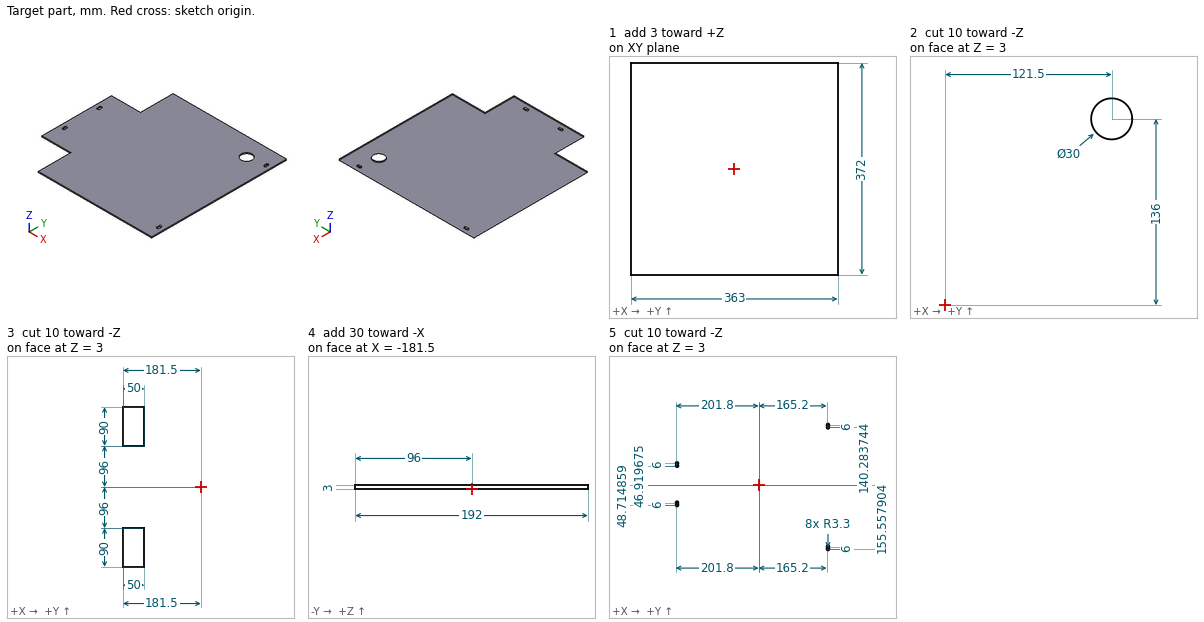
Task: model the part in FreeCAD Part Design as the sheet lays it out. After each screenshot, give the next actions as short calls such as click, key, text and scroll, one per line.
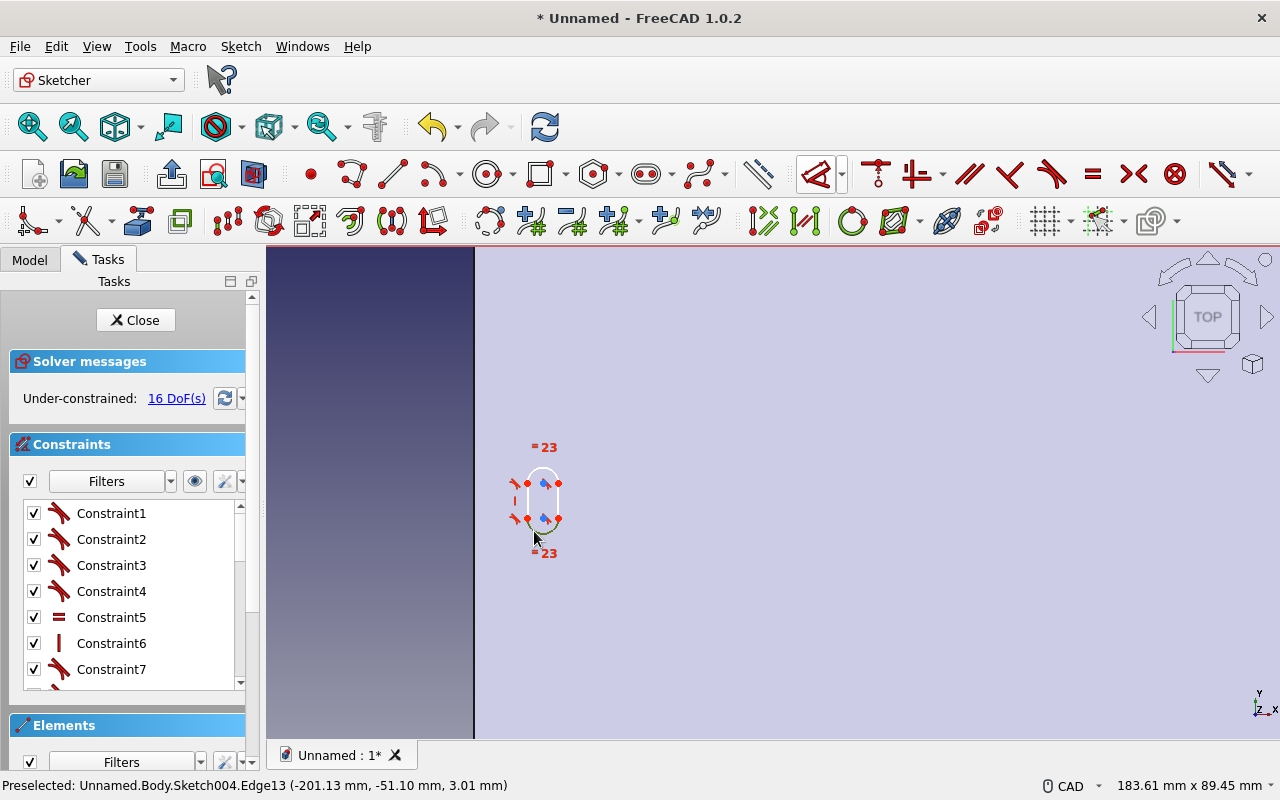
key(e)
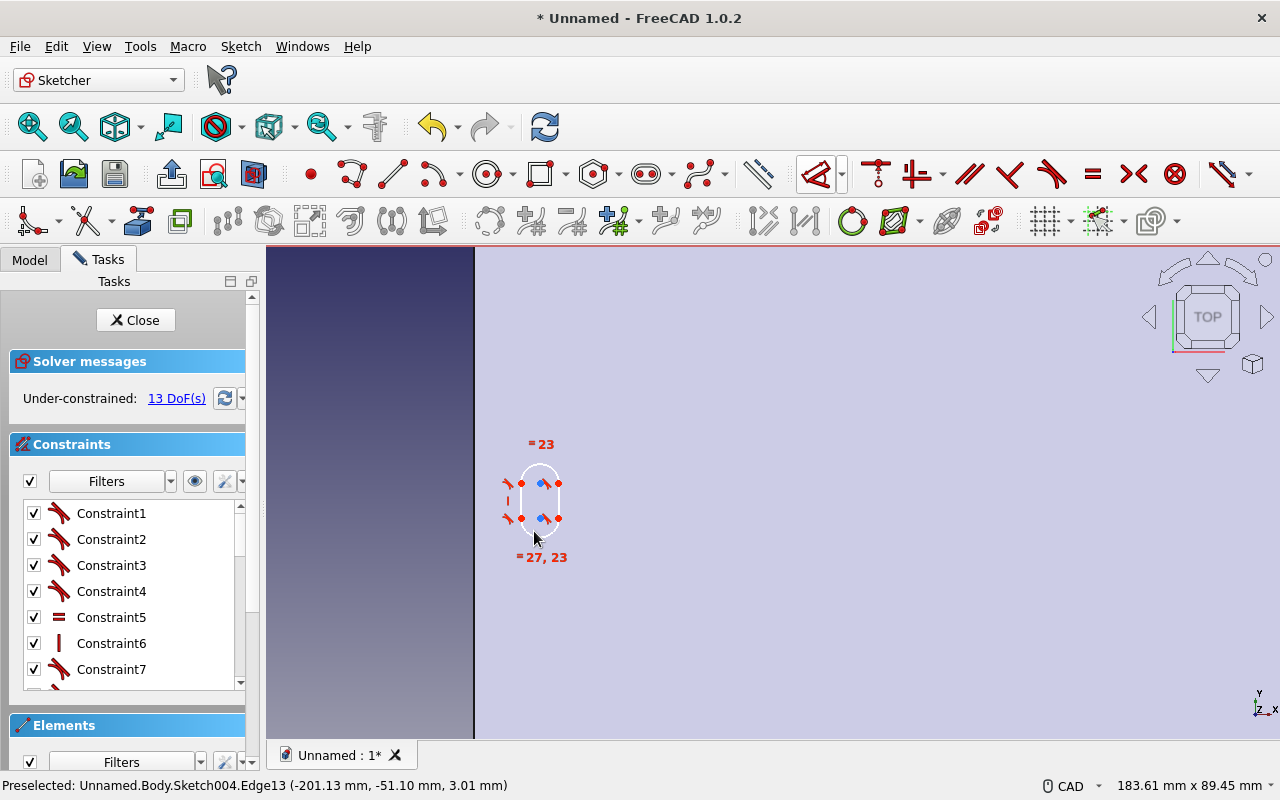
scroll(535, 536, down, 9)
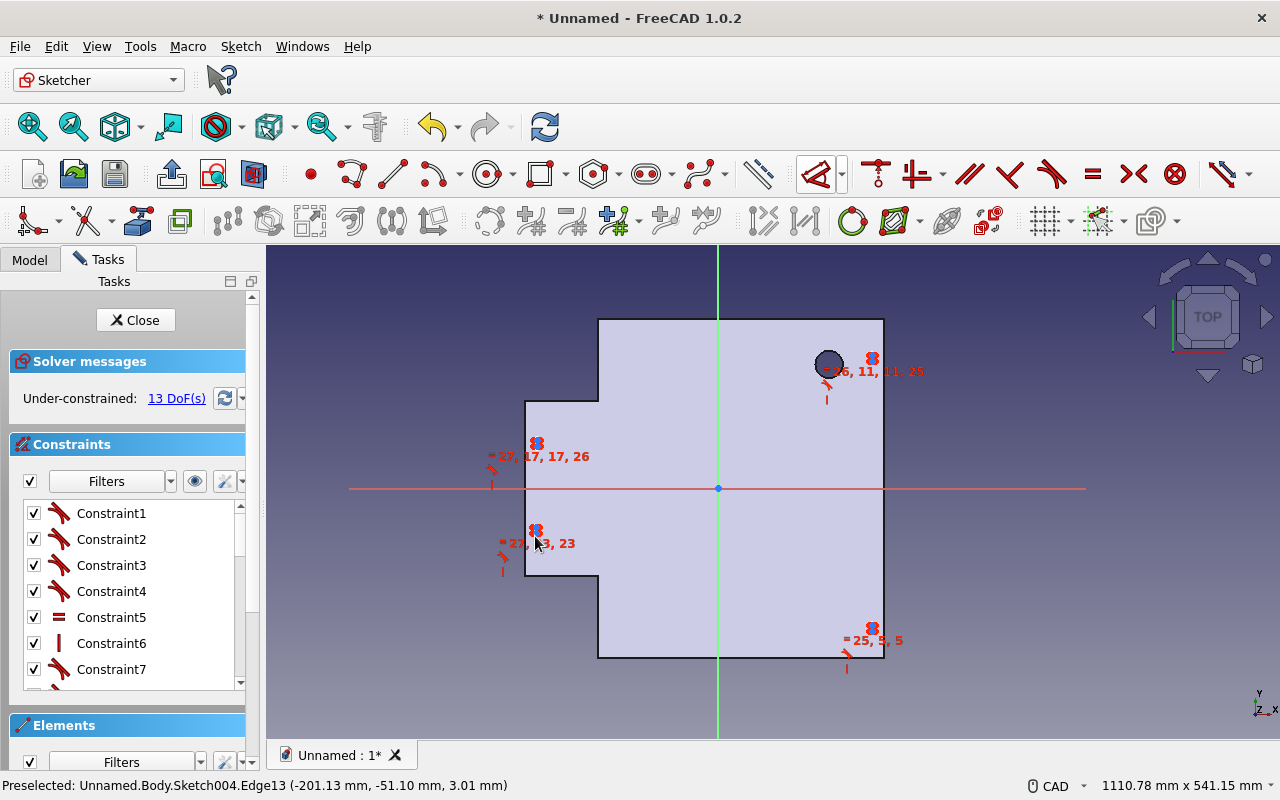
scroll(870, 634, up, 13)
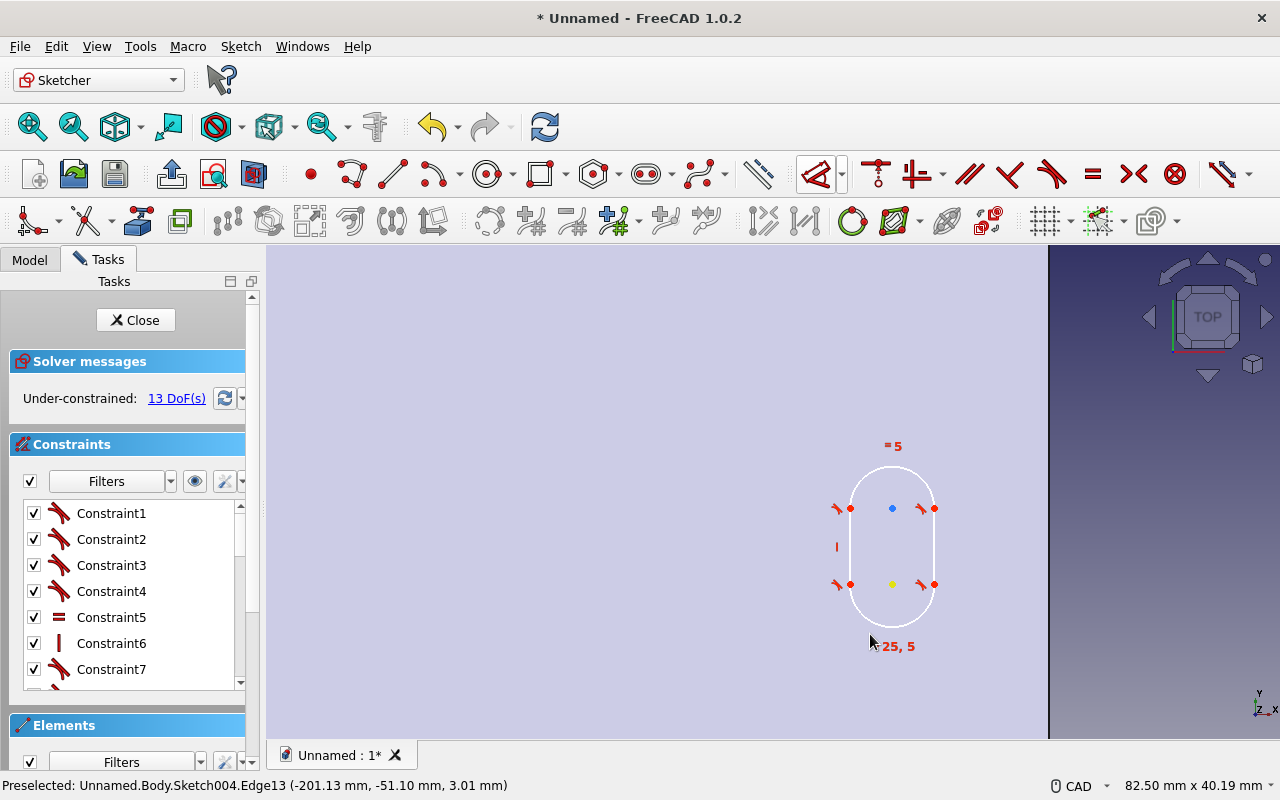
click(867, 619)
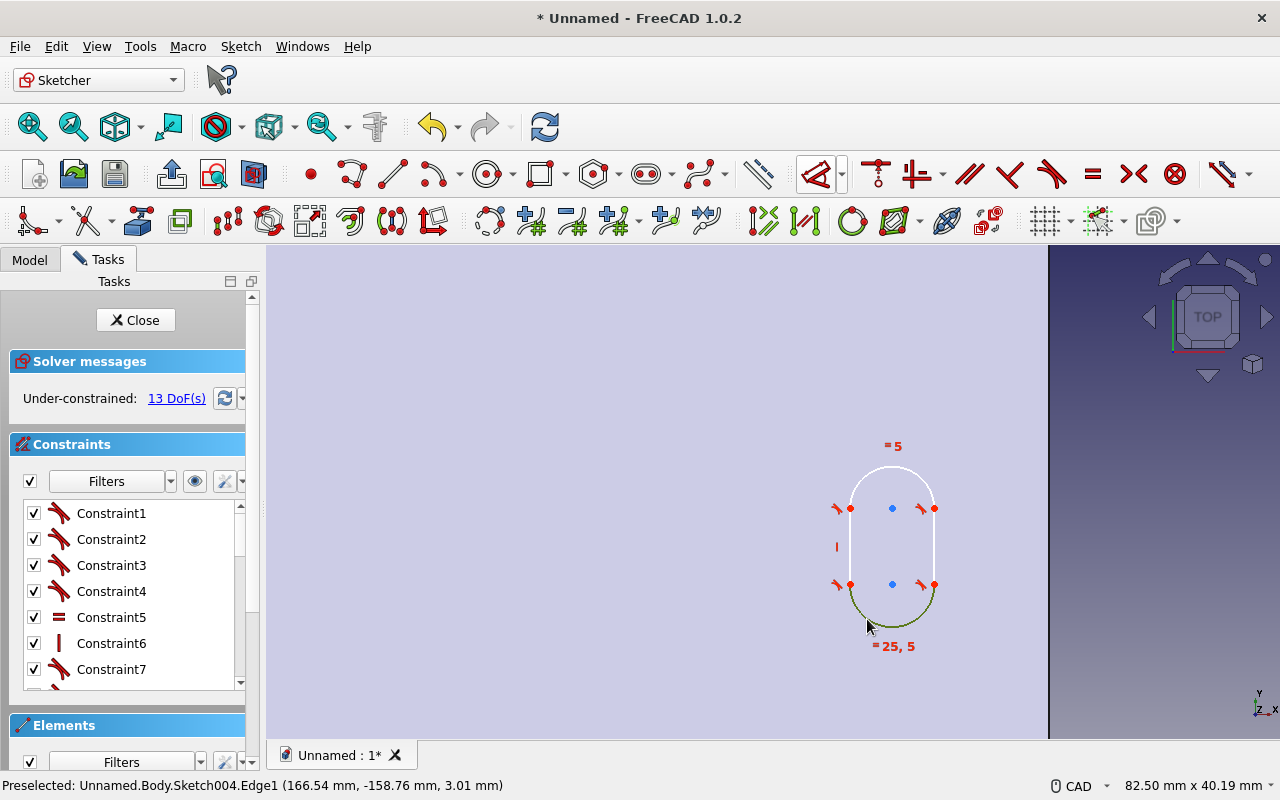
key(k)
key(r)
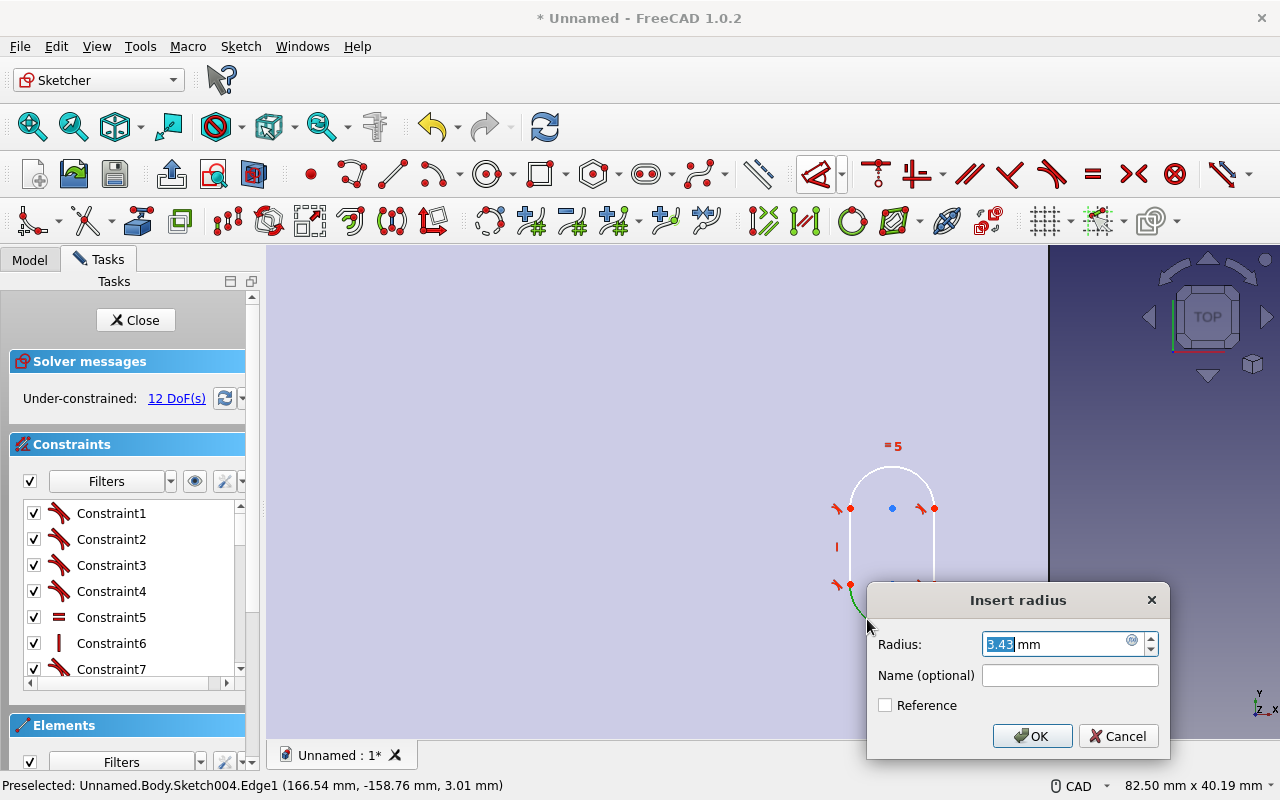
text(3.3)
key(Return)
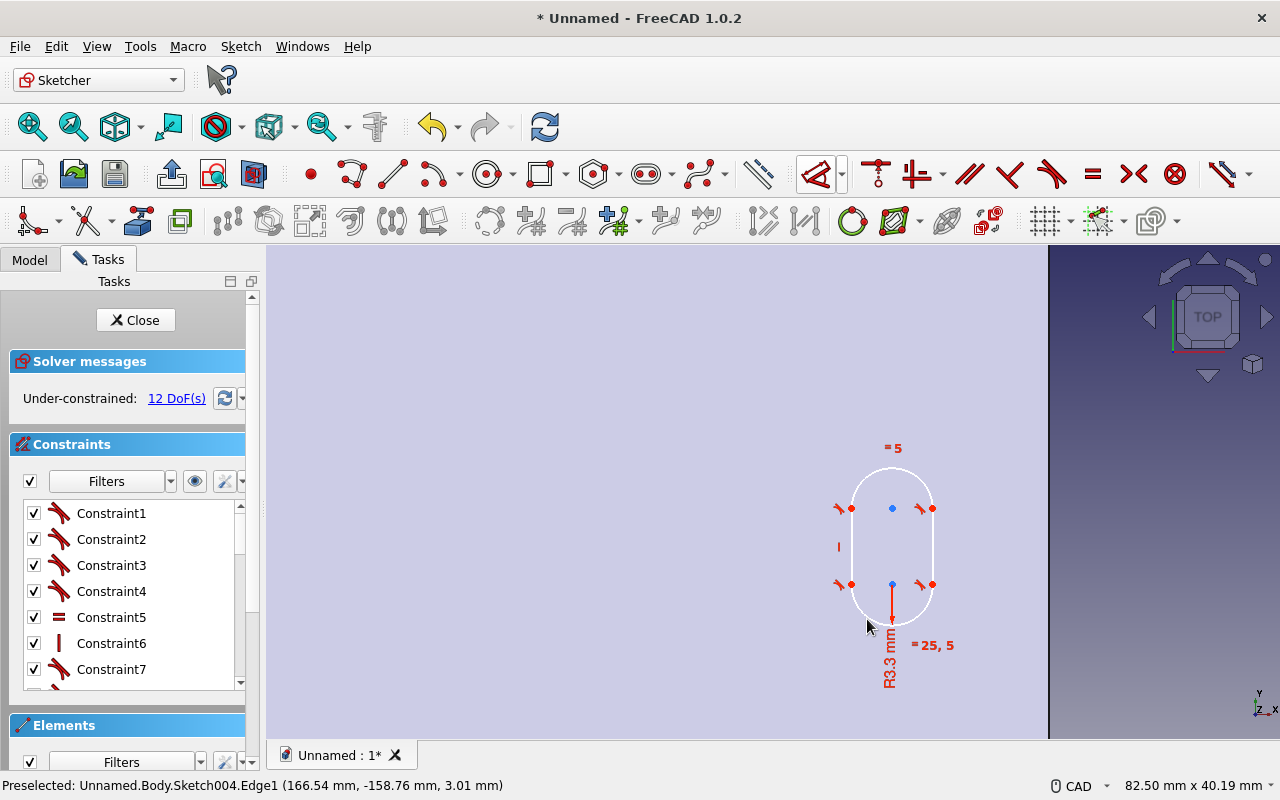
click(852, 562)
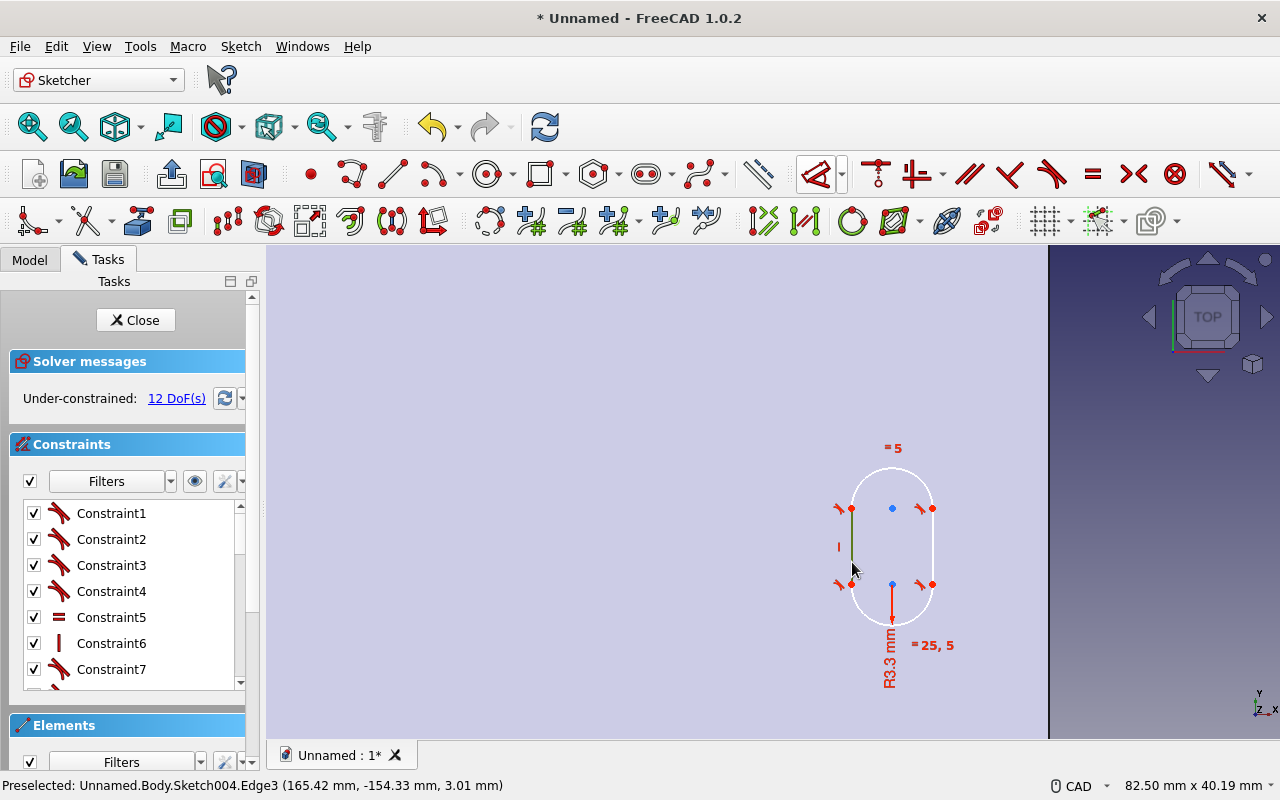
click(842, 174)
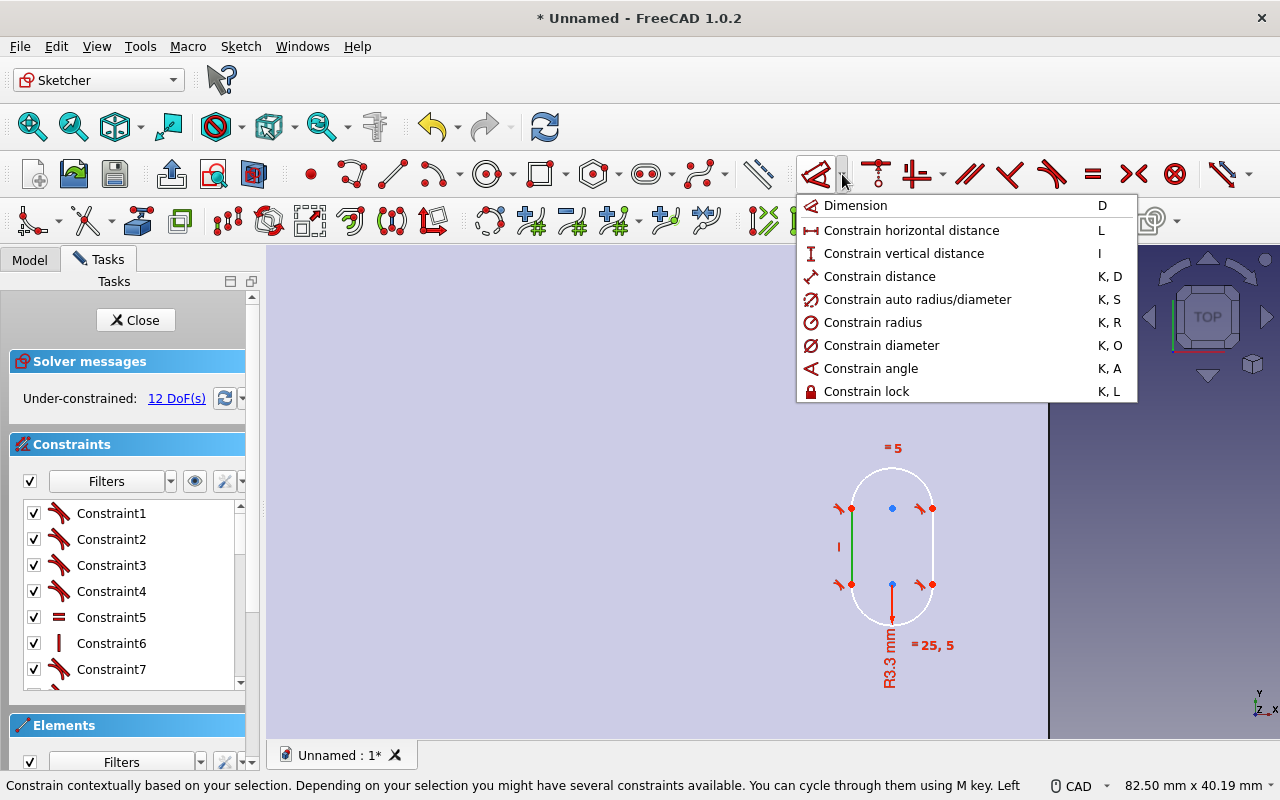
click(967, 254)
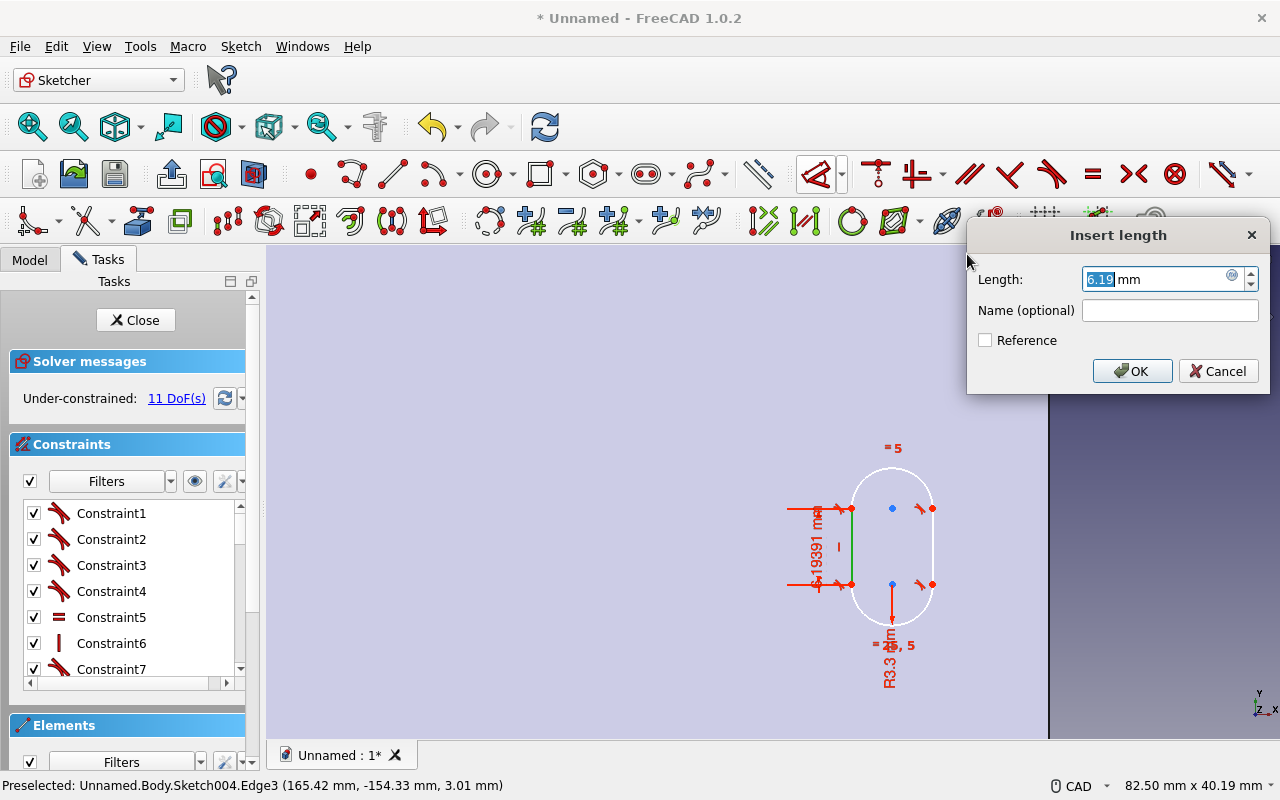
text(6)
key(Return)